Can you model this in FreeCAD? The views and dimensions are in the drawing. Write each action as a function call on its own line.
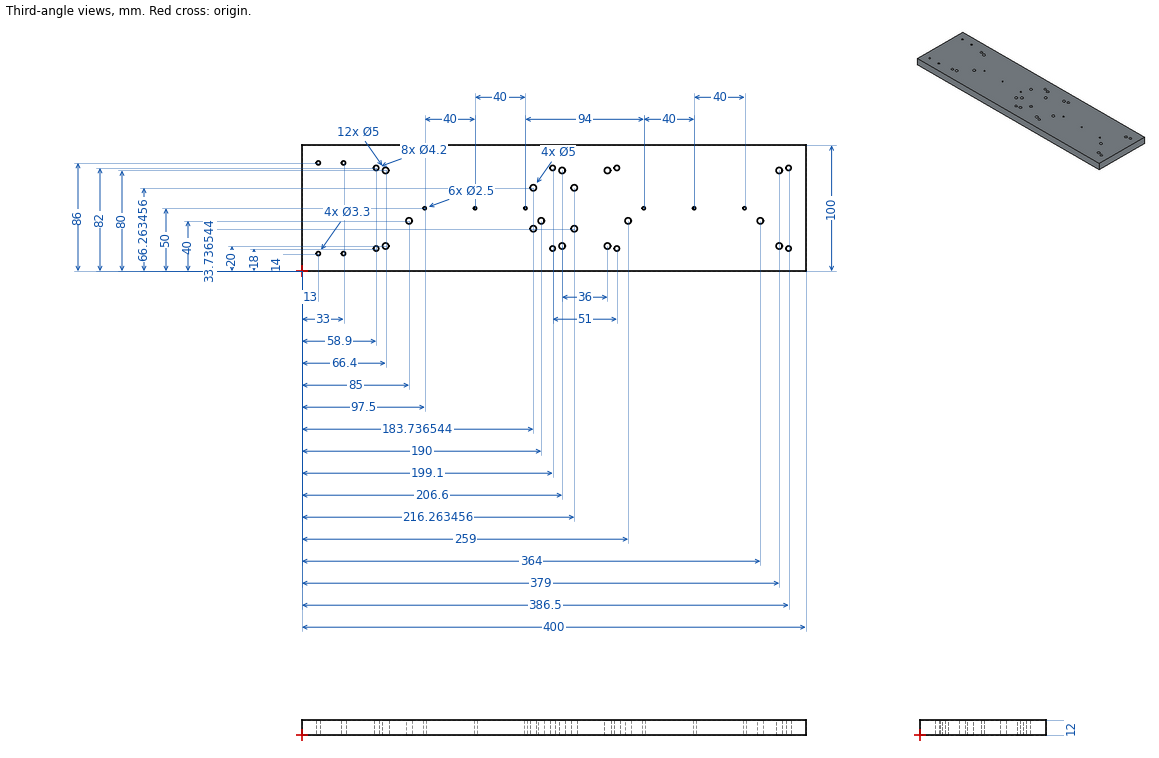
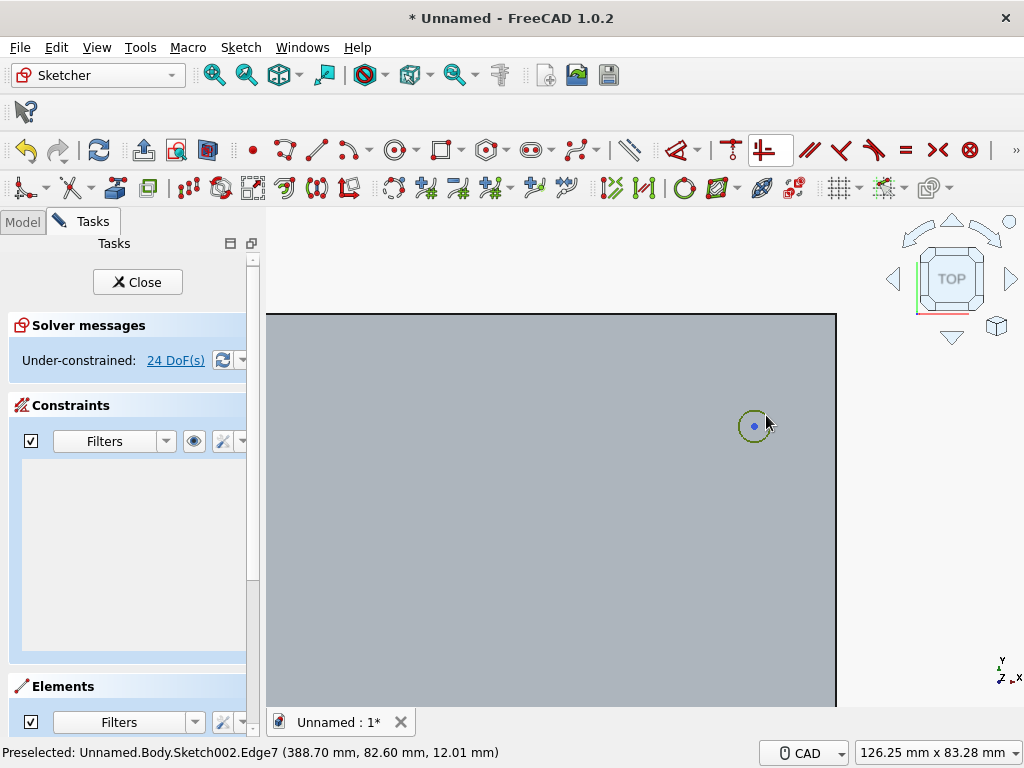
scroll(770, 416, down, 9)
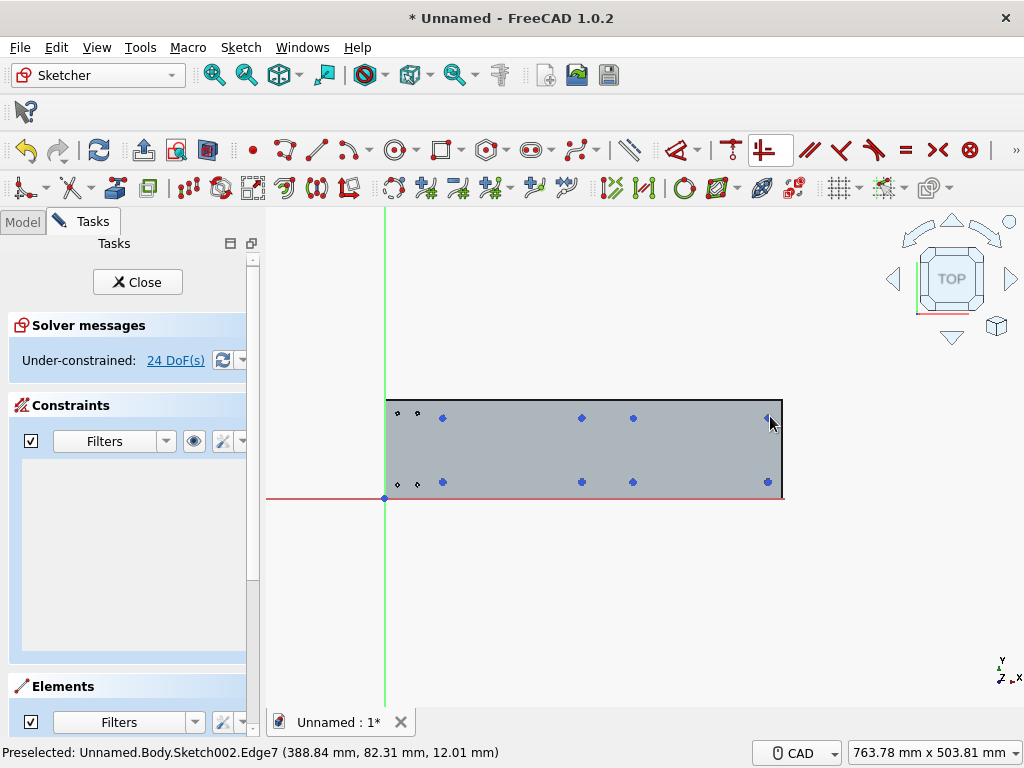
scroll(770, 480, up, 8)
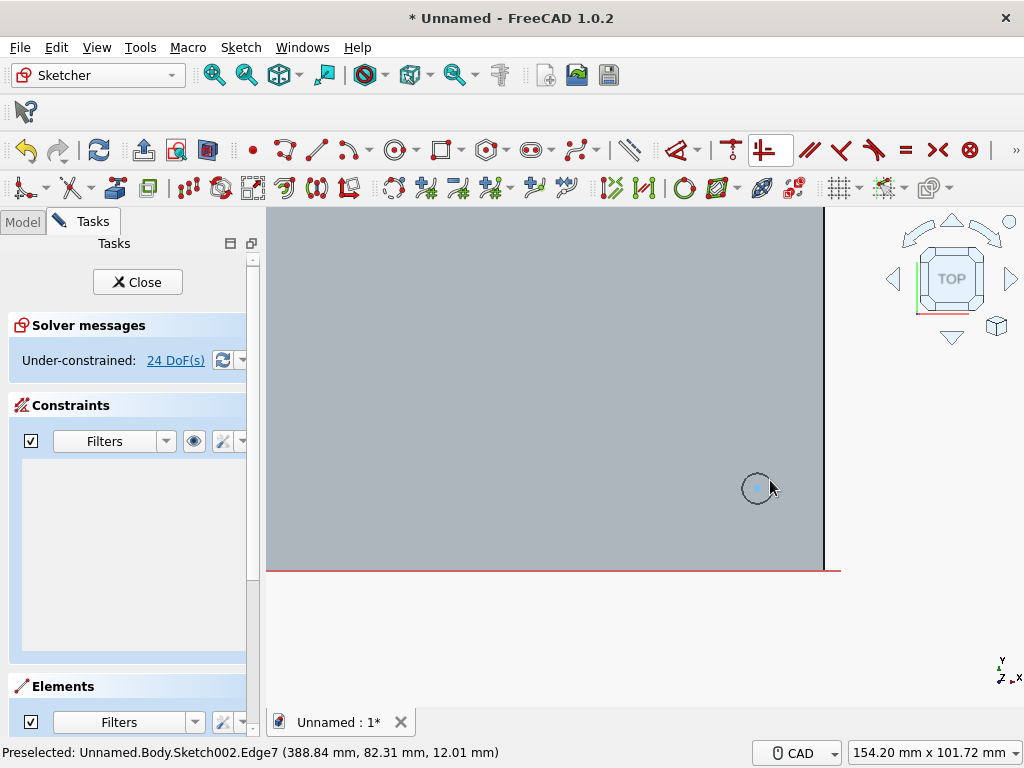
click(768, 478)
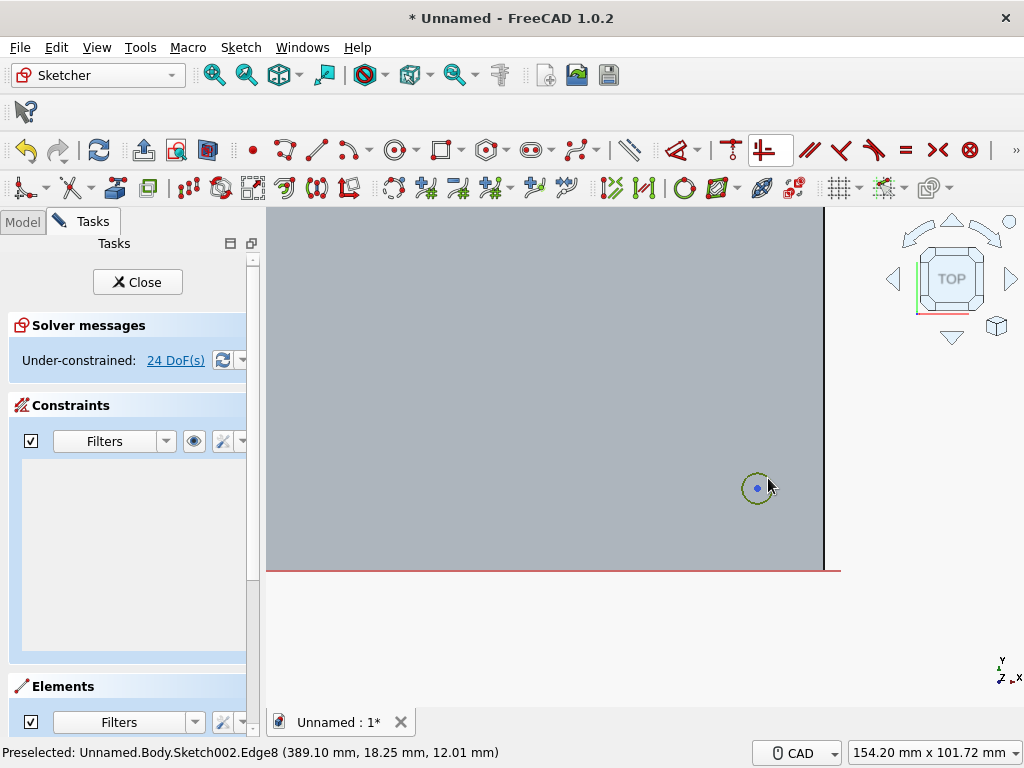
click(906, 150)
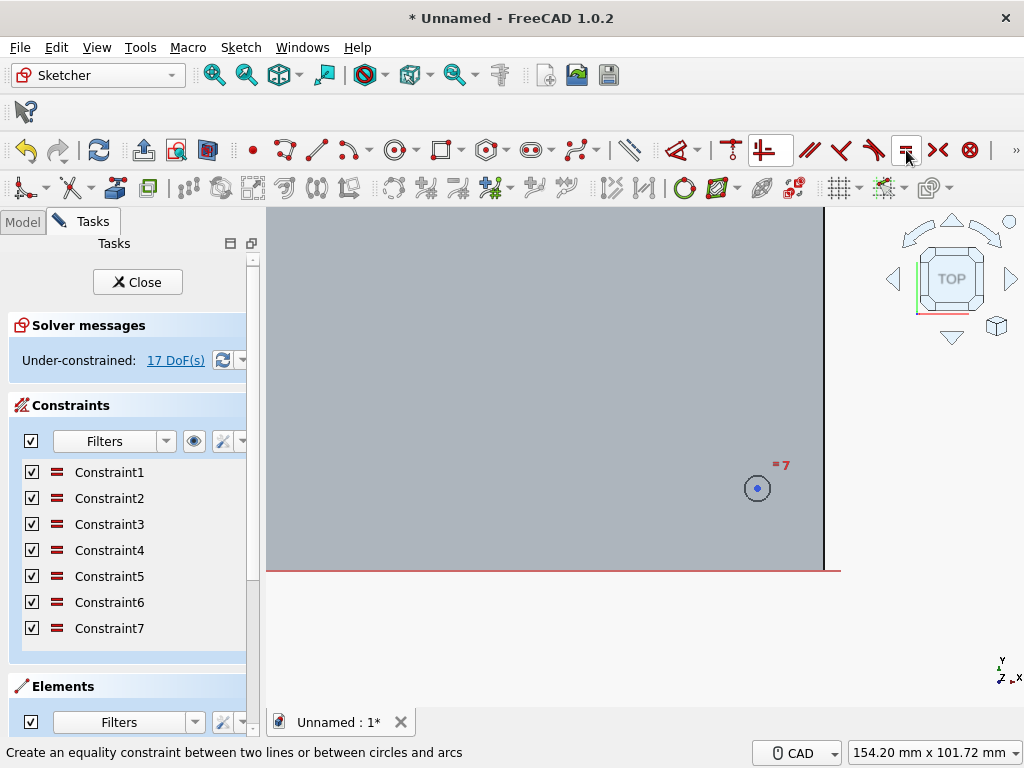
scroll(770, 480, down, 8)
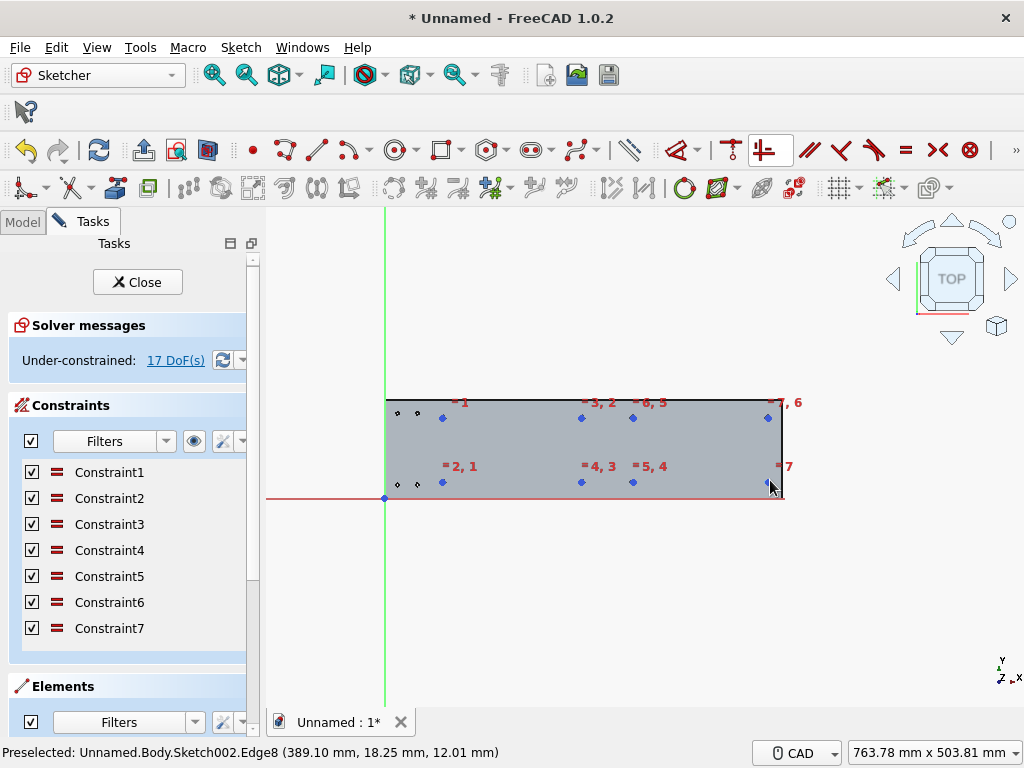
click(443, 418)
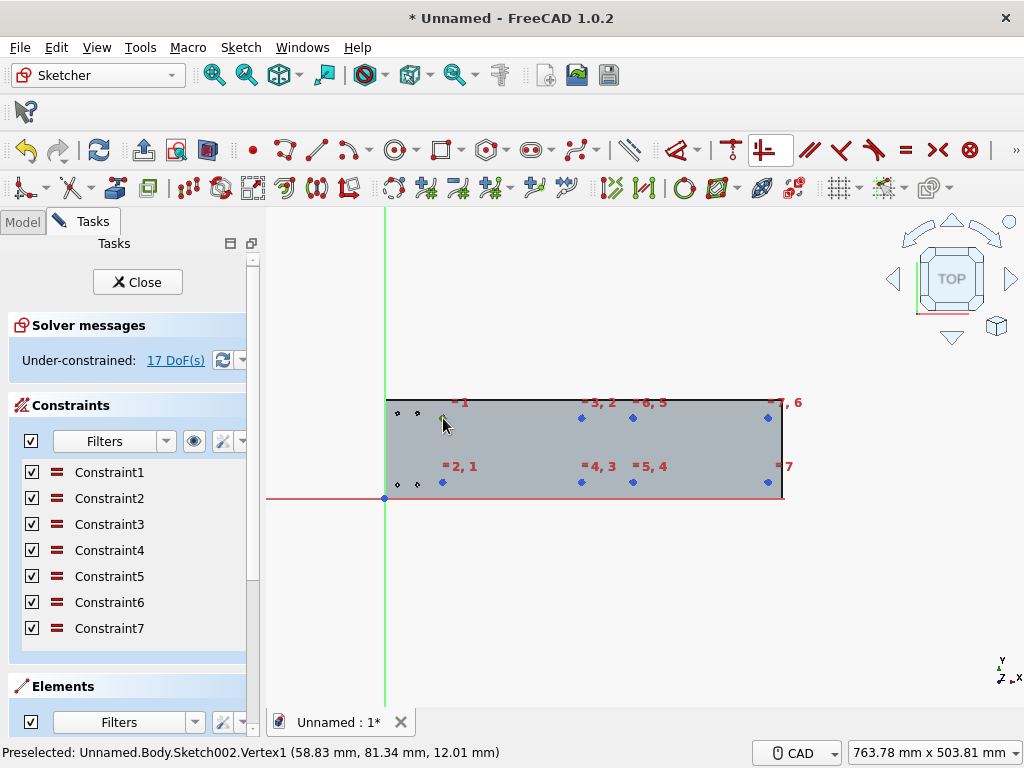
click(443, 482)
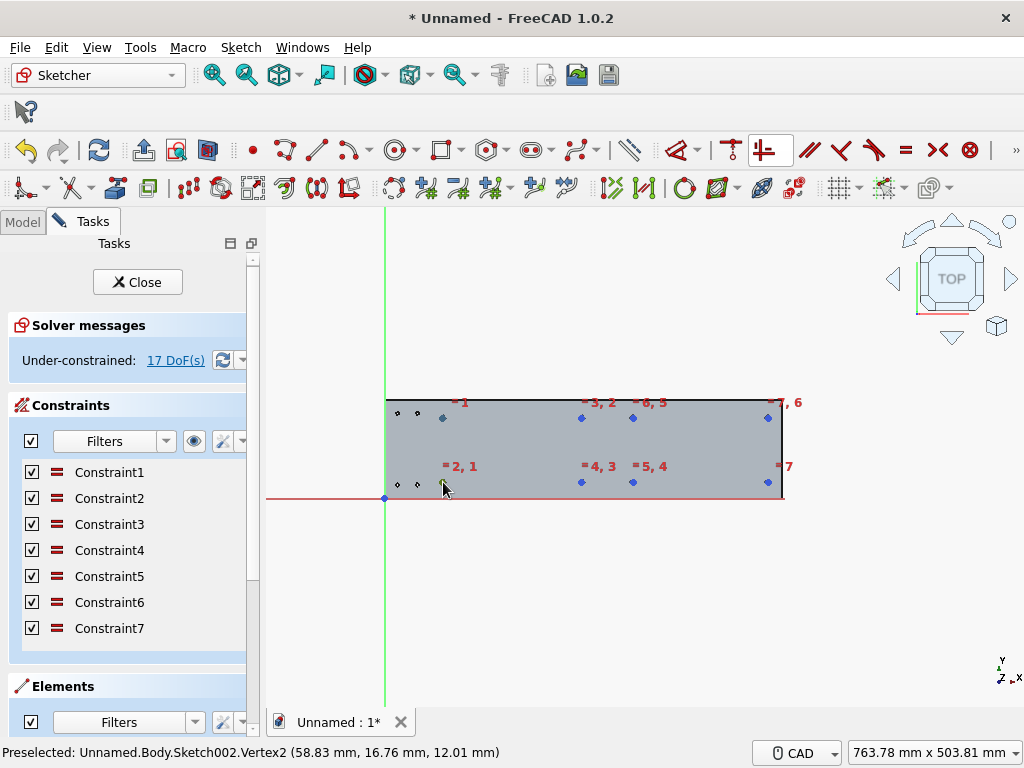
click(788, 150)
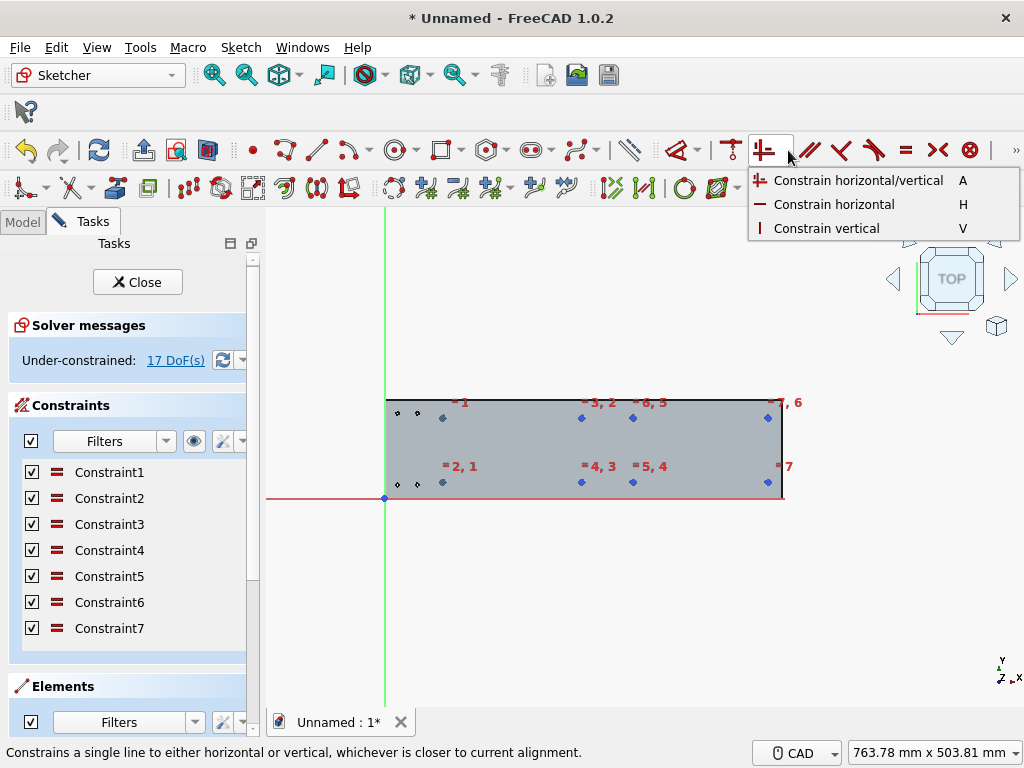
click(884, 228)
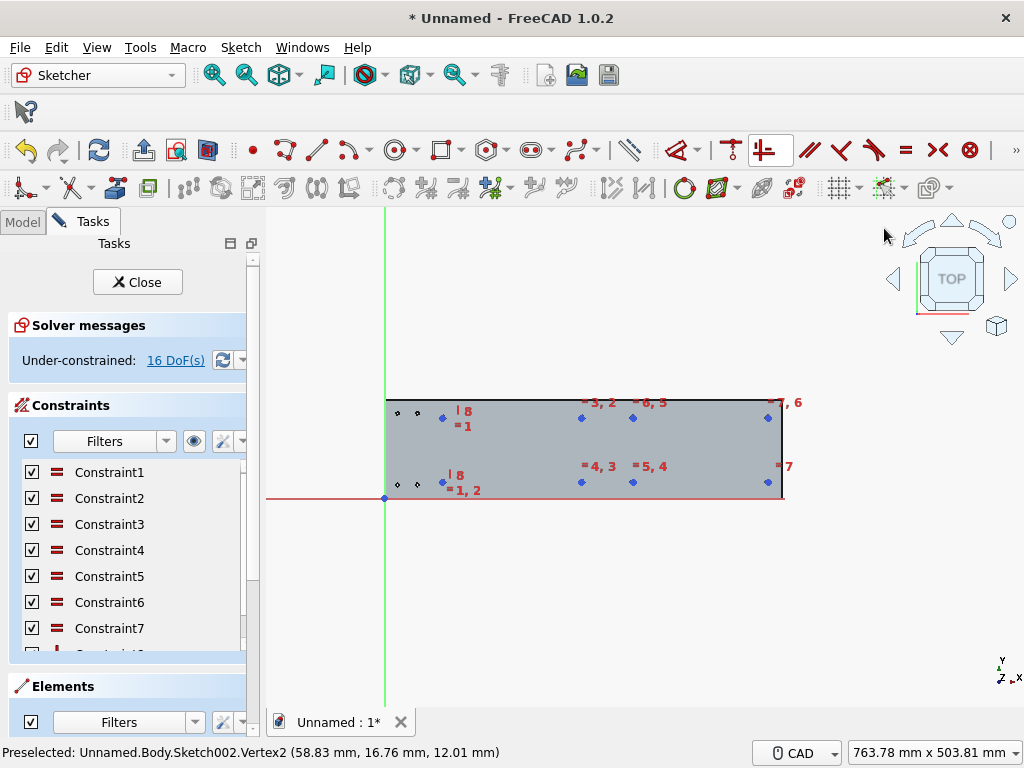
click(443, 418)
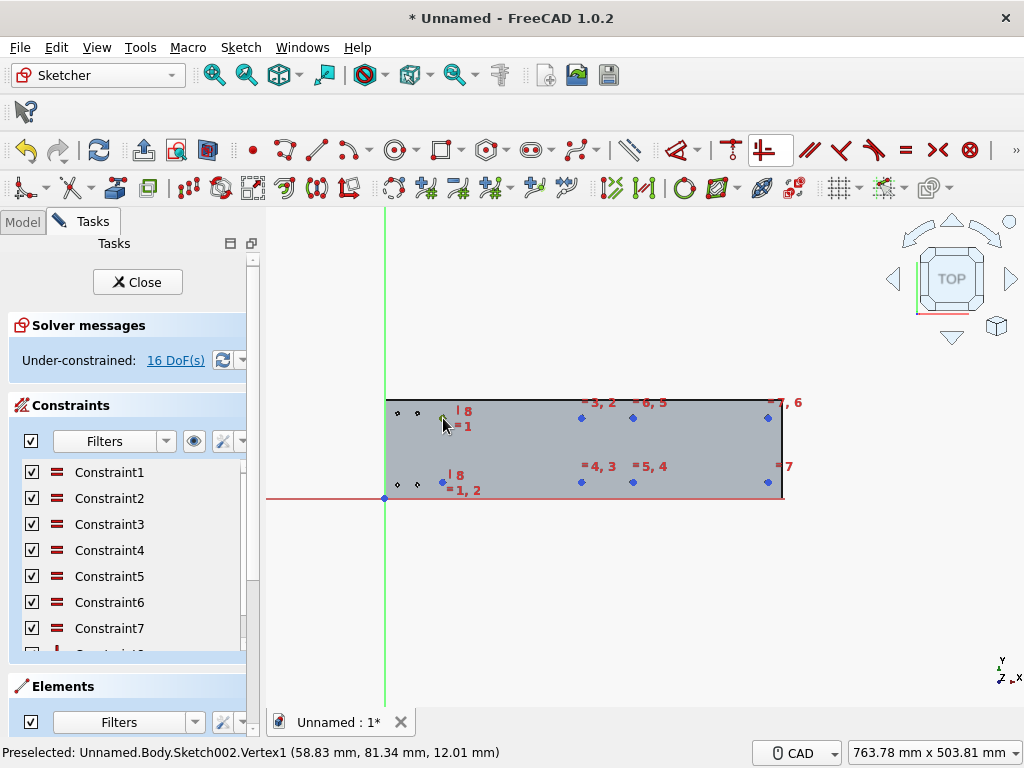
click(582, 418)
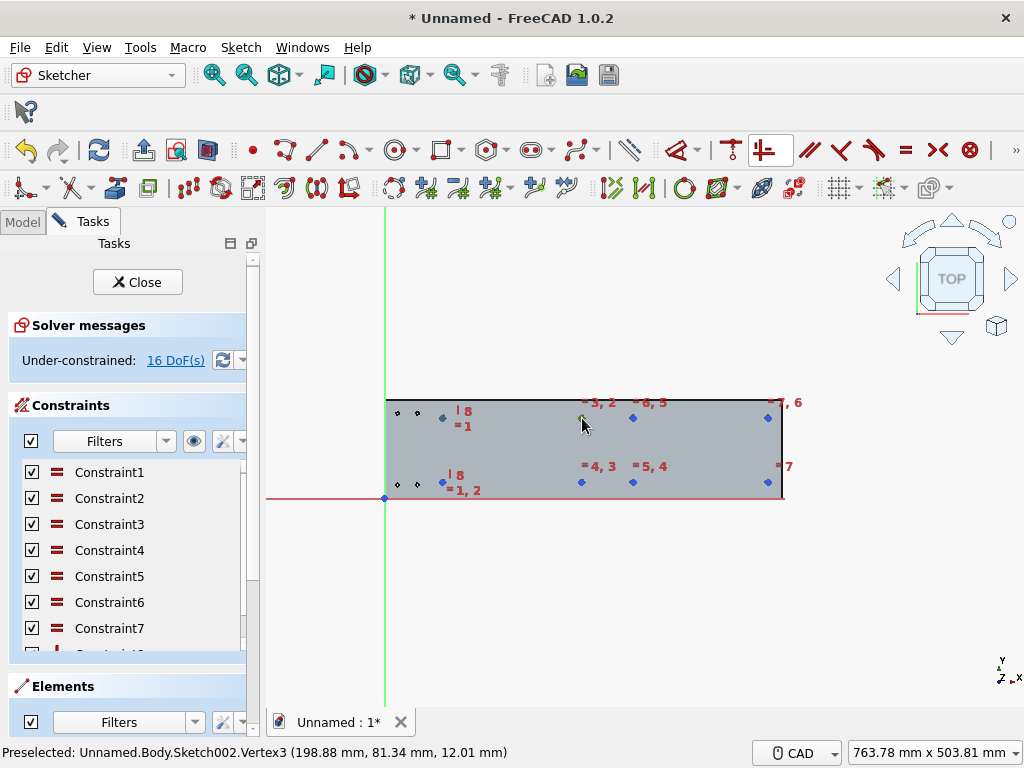
click(788, 150)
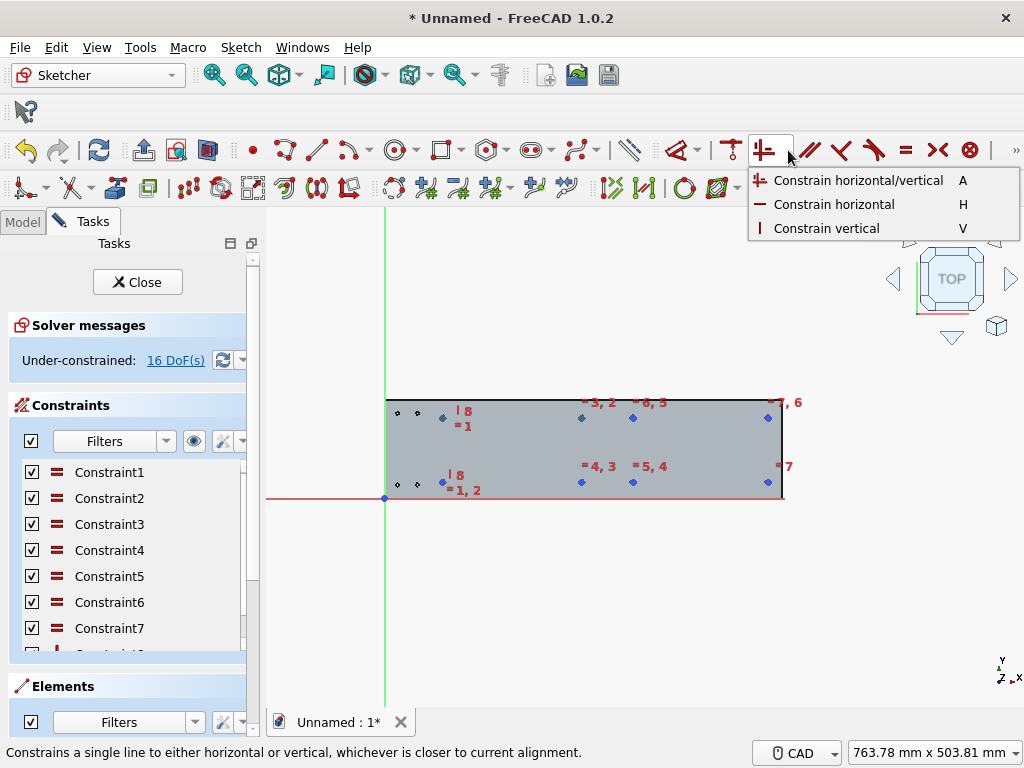
click(884, 204)